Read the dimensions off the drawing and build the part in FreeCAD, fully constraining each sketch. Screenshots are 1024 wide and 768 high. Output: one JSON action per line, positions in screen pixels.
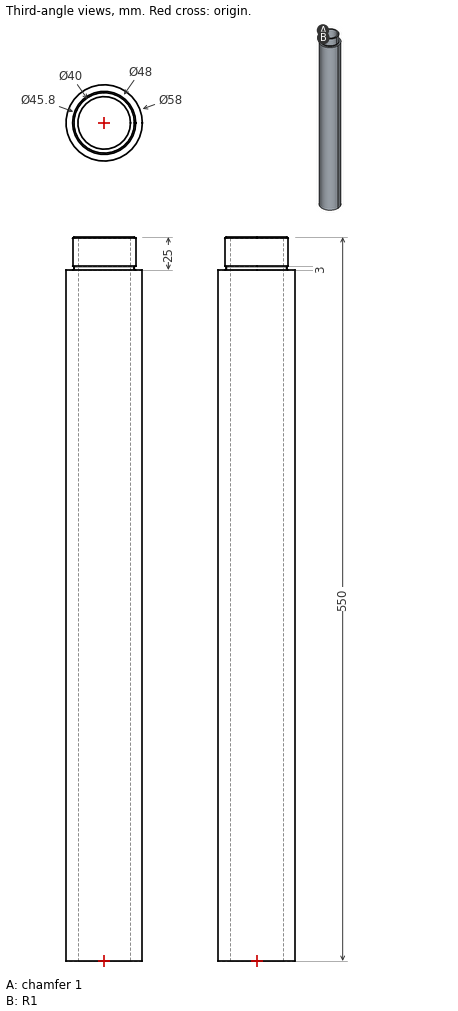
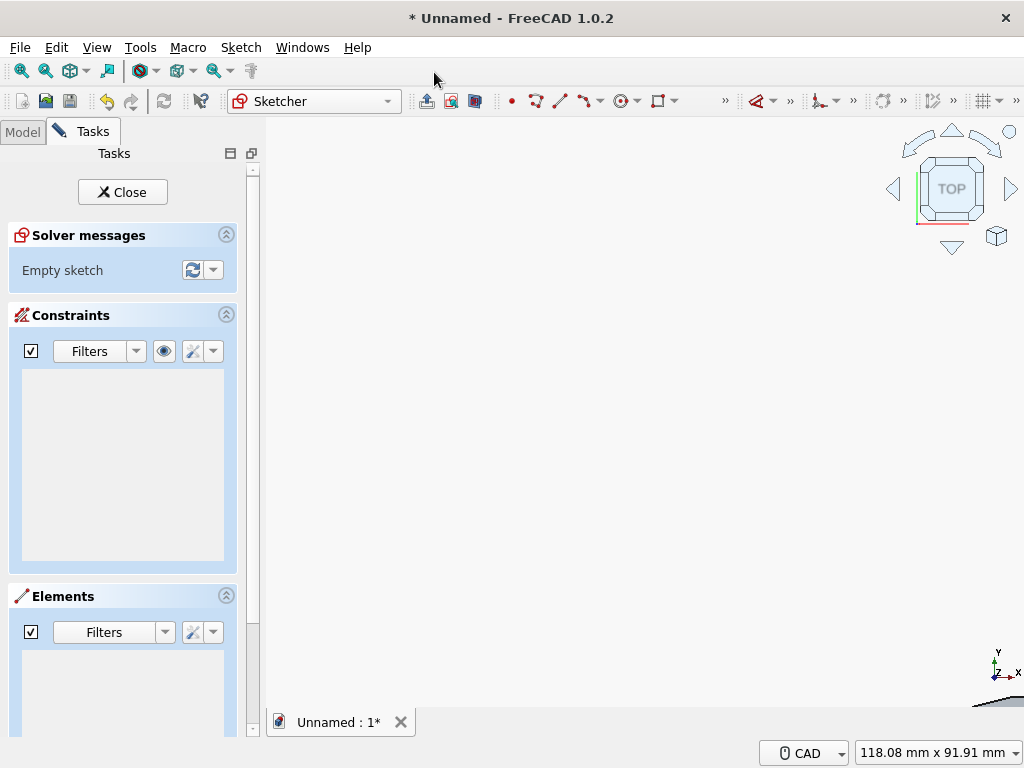
{"action": "left_click", "coordinate": [476, 102]}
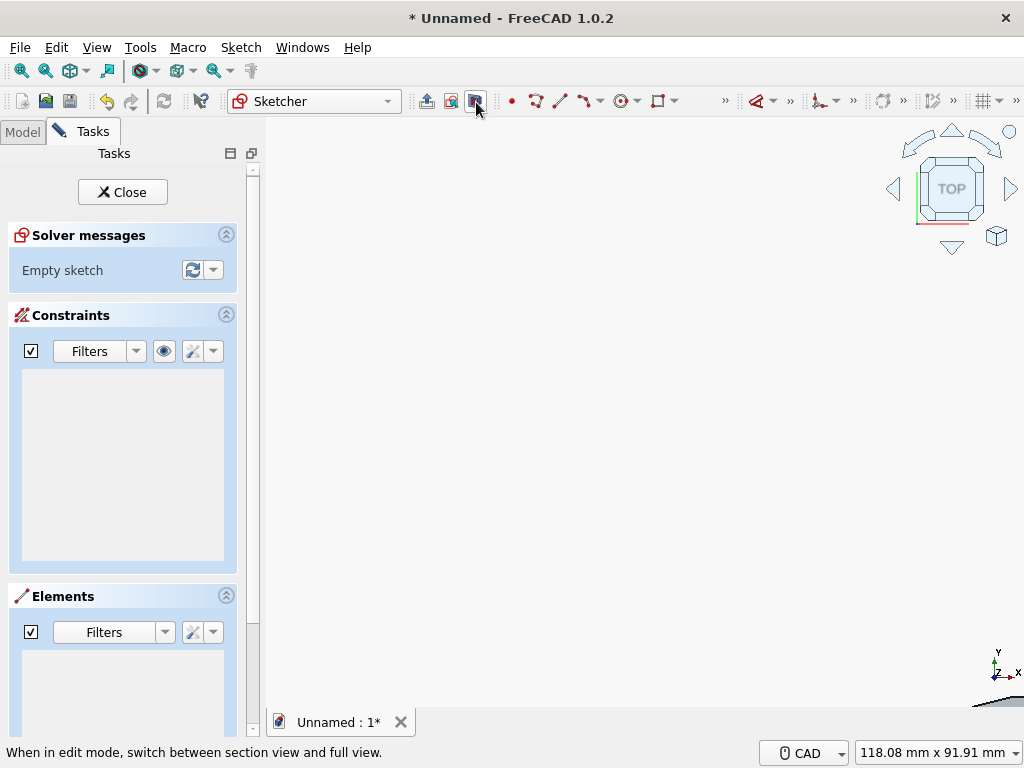
{"action": "scroll", "coordinate": [576, 412], "scroll_direction": "down", "scroll_amount": 5}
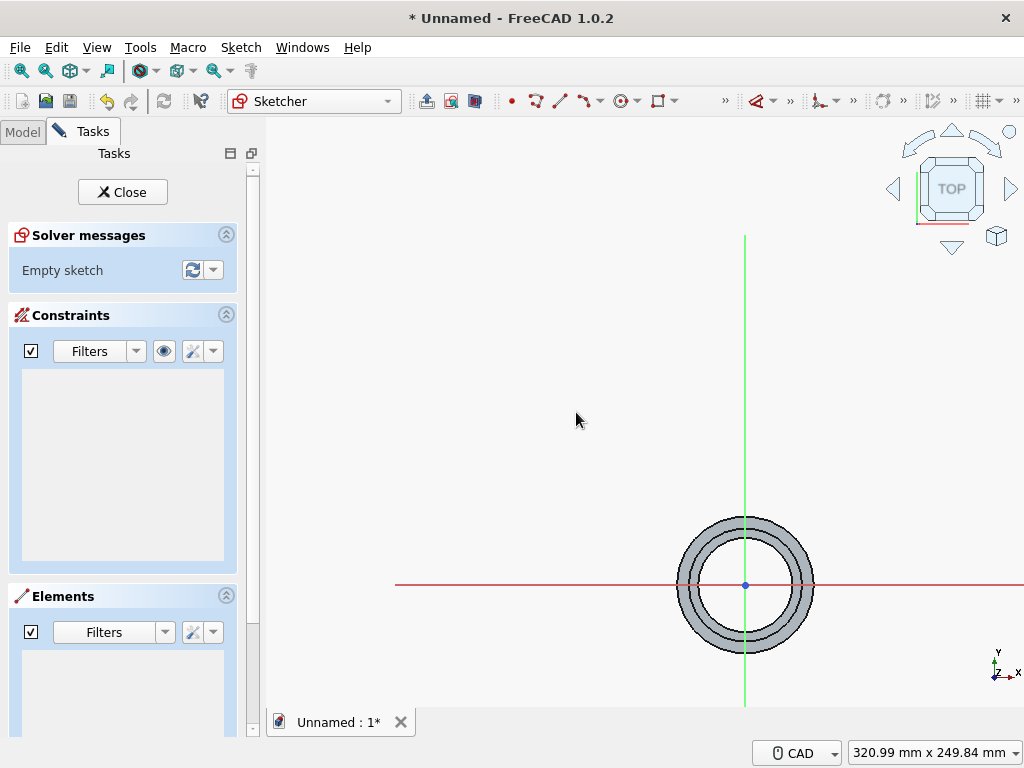
{"action": "scroll", "coordinate": [818, 660], "scroll_direction": "up", "scroll_amount": 6}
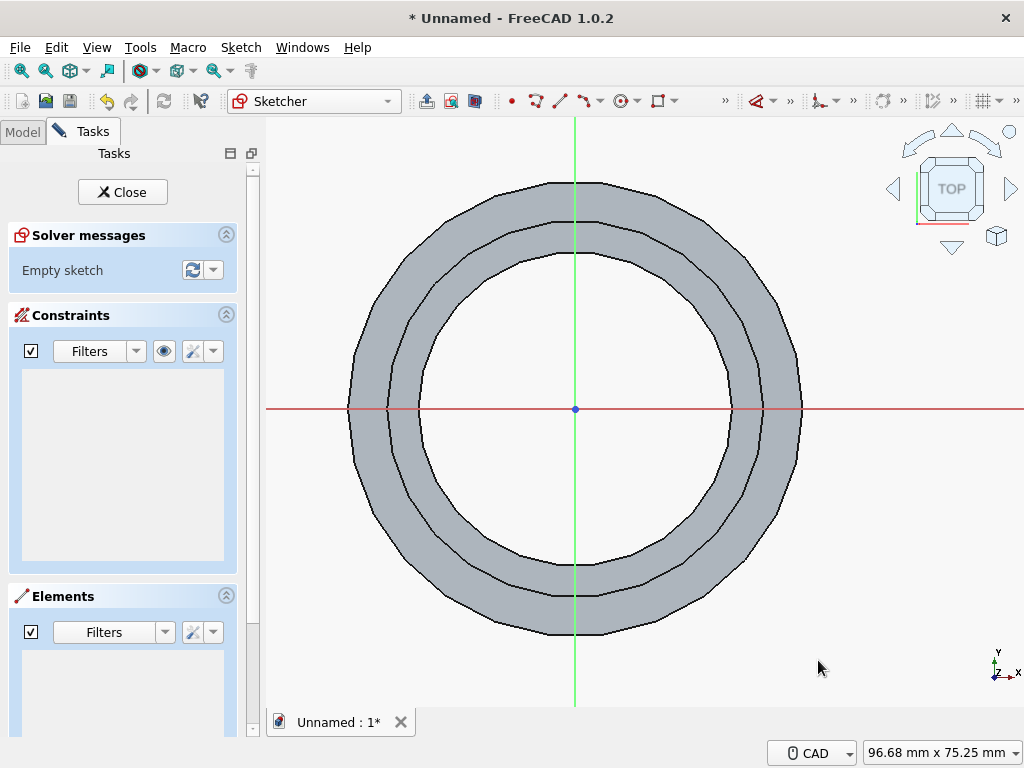
{"action": "left_click", "coordinate": [622, 102]}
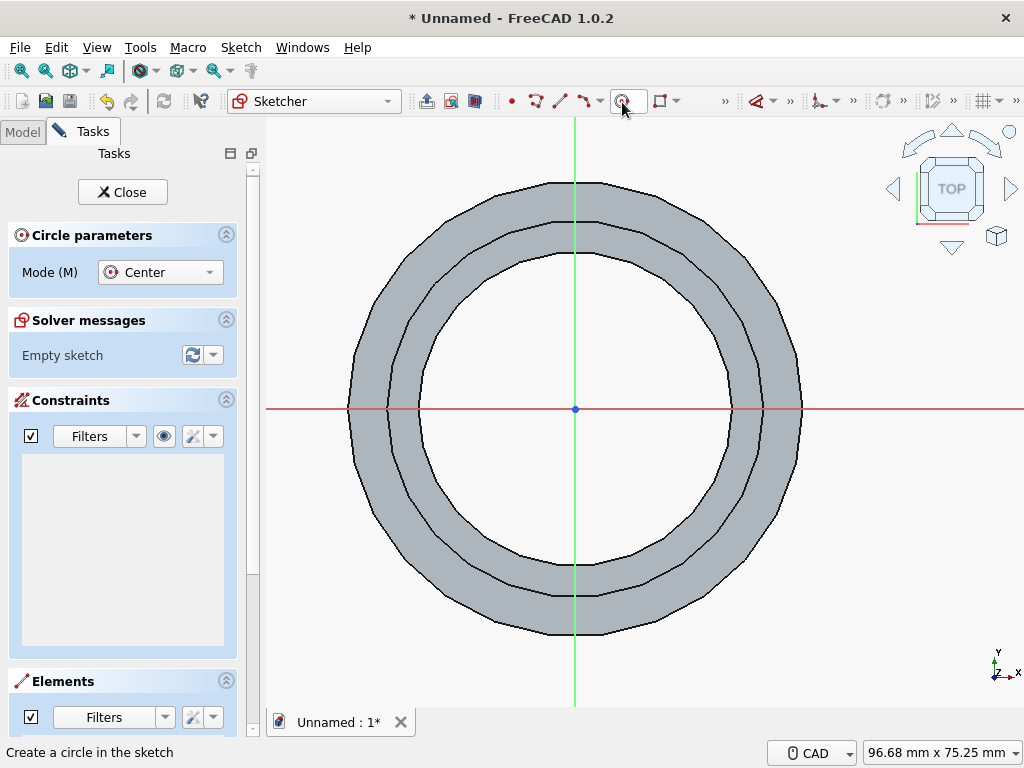
{"action": "left_click", "coordinate": [575, 409]}
{"action": "mouse_move", "coordinate": [708, 276]}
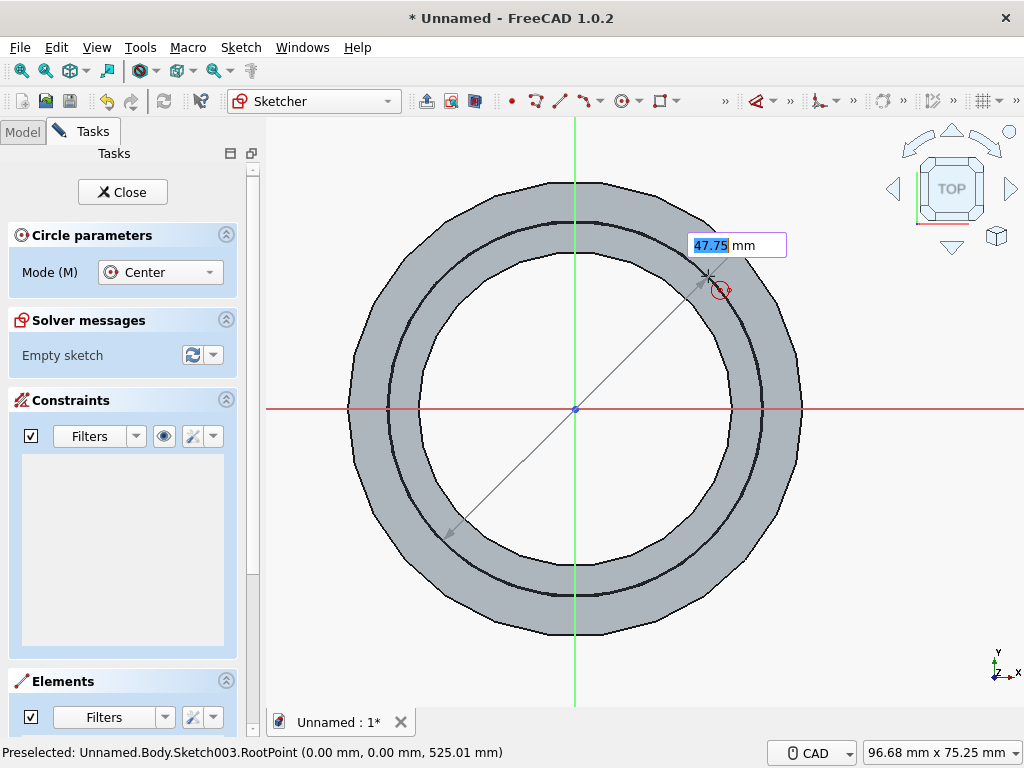
{"action": "type", "text": "48"}
{"action": "key", "text": "Return"}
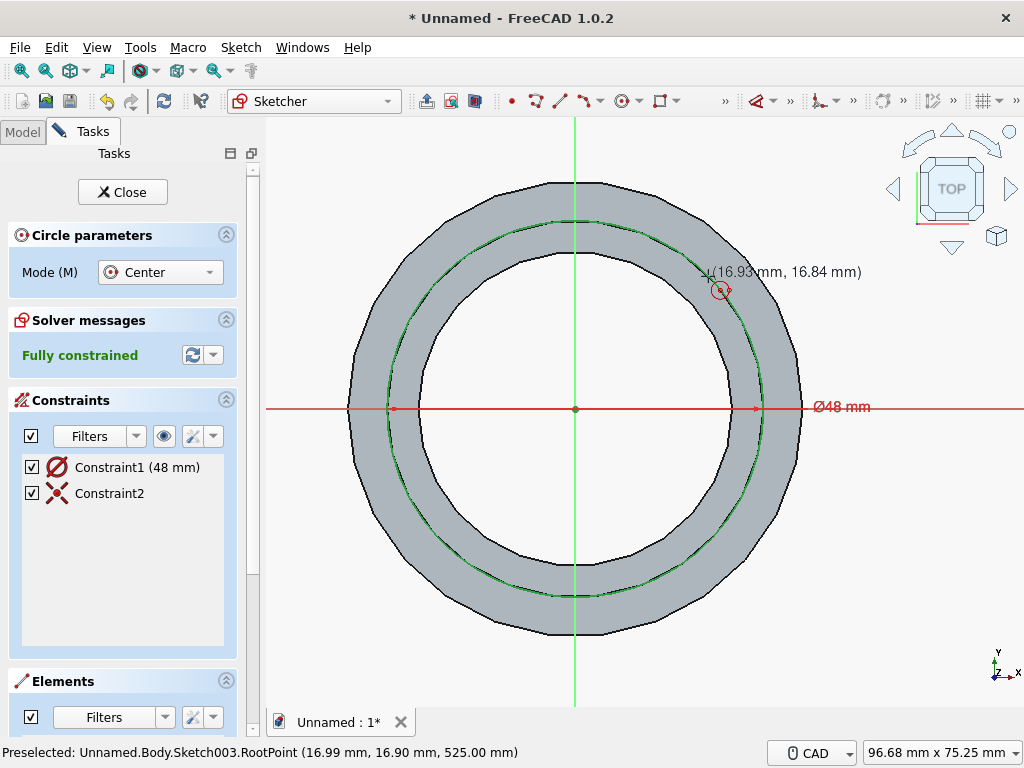
{"action": "left_click", "coordinate": [575, 409]}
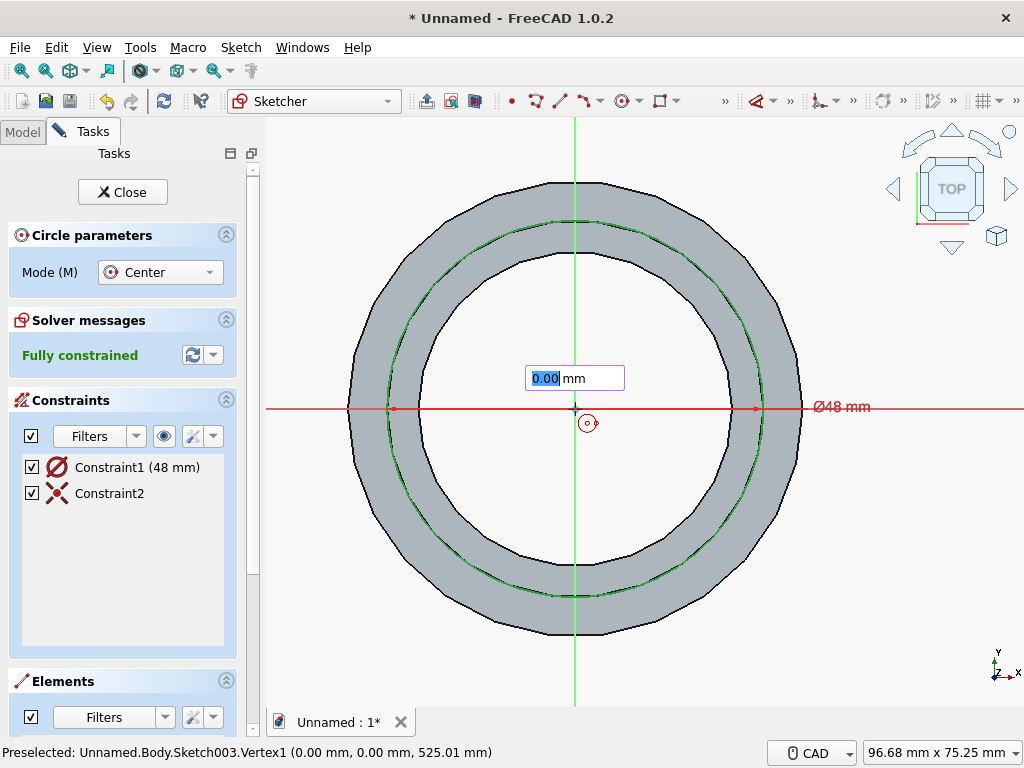
{"action": "scroll", "coordinate": [702, 282], "scroll_direction": "up", "scroll_amount": 4}
{"action": "mouse_move", "coordinate": [702, 282]}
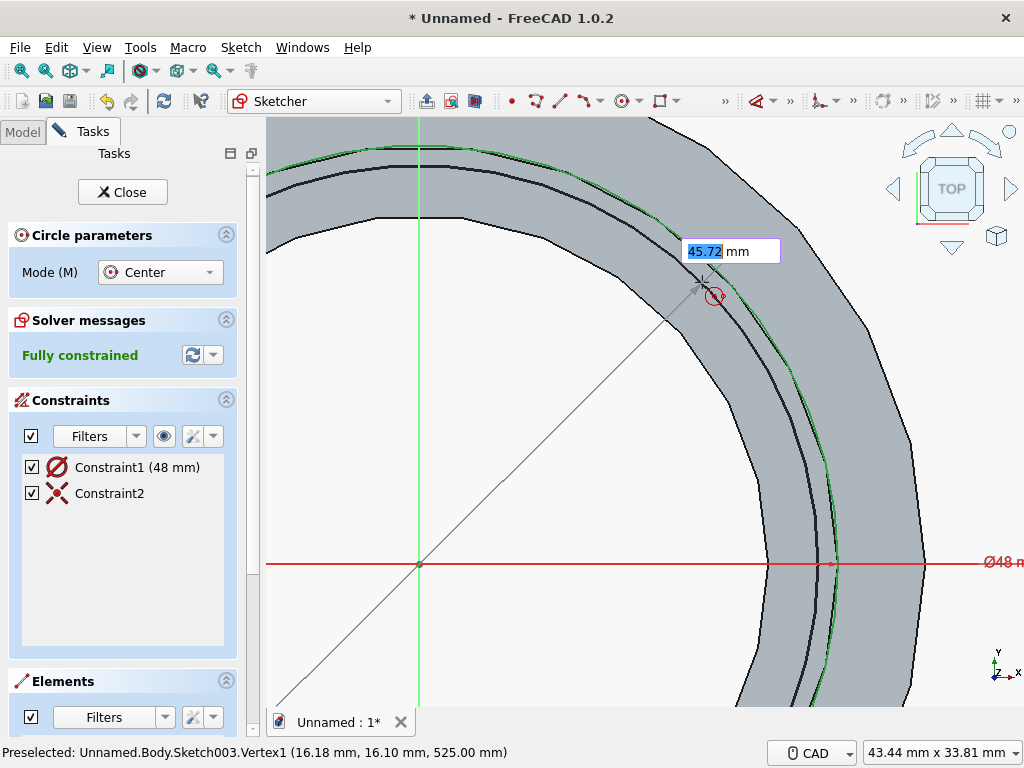
{"action": "type", "text": "45.8"}
{"action": "key", "text": "Return"}
{"action": "key", "text": "Escape"}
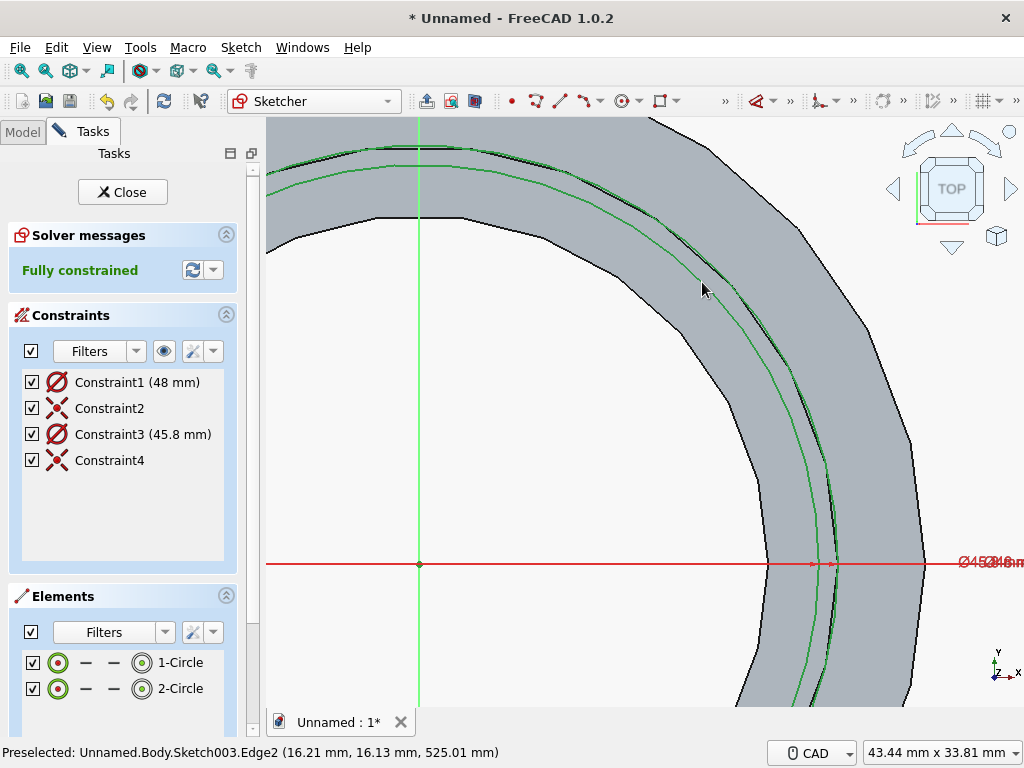
{"action": "left_click", "coordinate": [123, 192]}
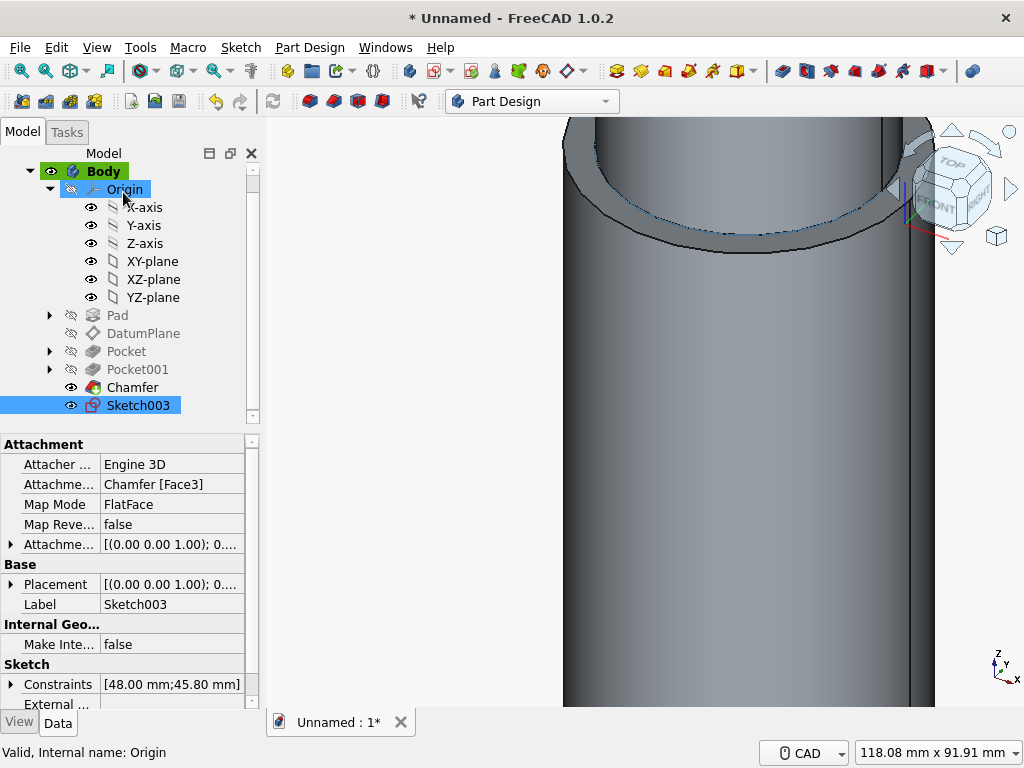
{"action": "left_click", "coordinate": [784, 72]}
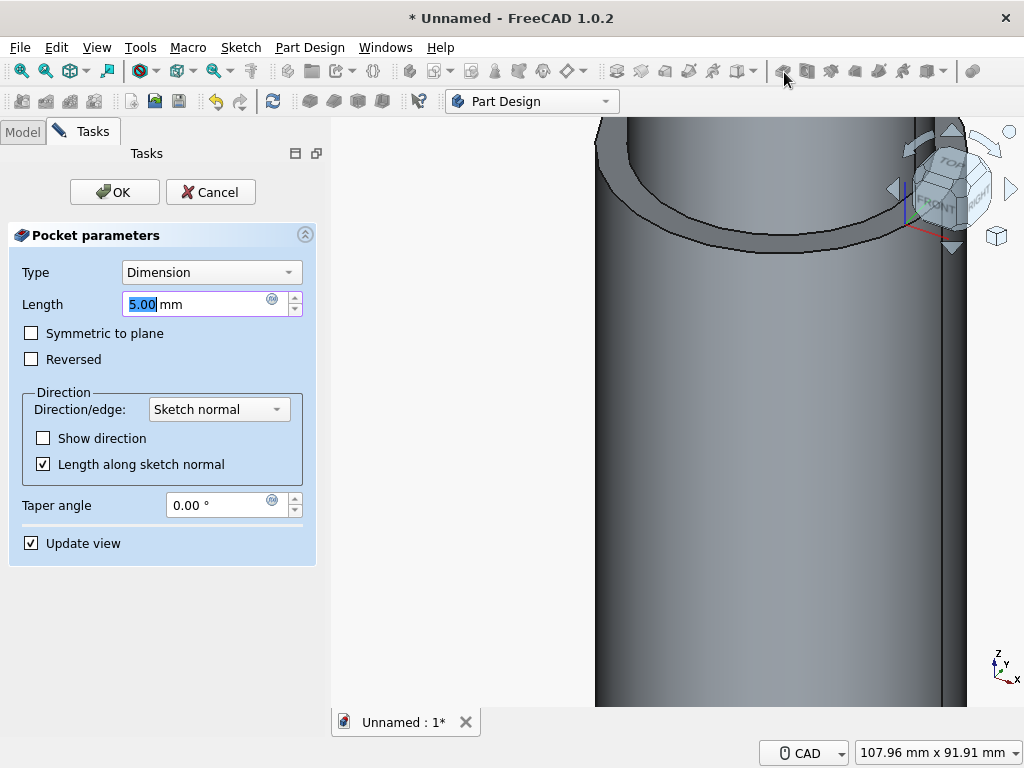
{"action": "type", "text": "3"}
{"action": "key", "text": "Tab"}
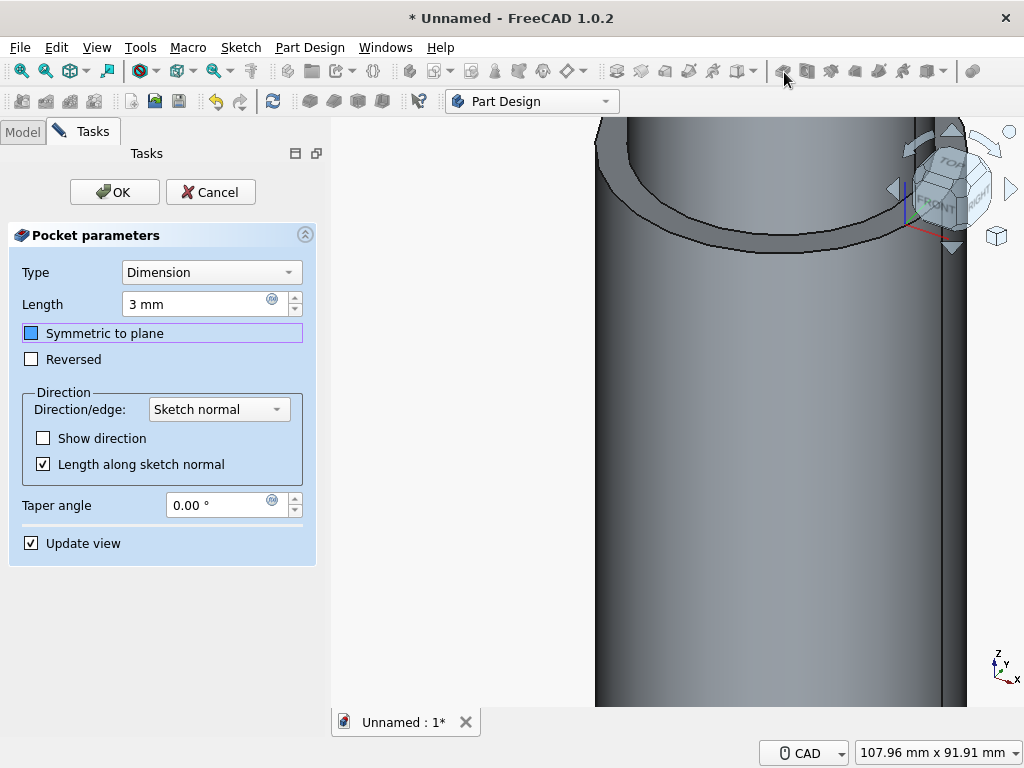
{"action": "left_click", "coordinate": [30, 359]}